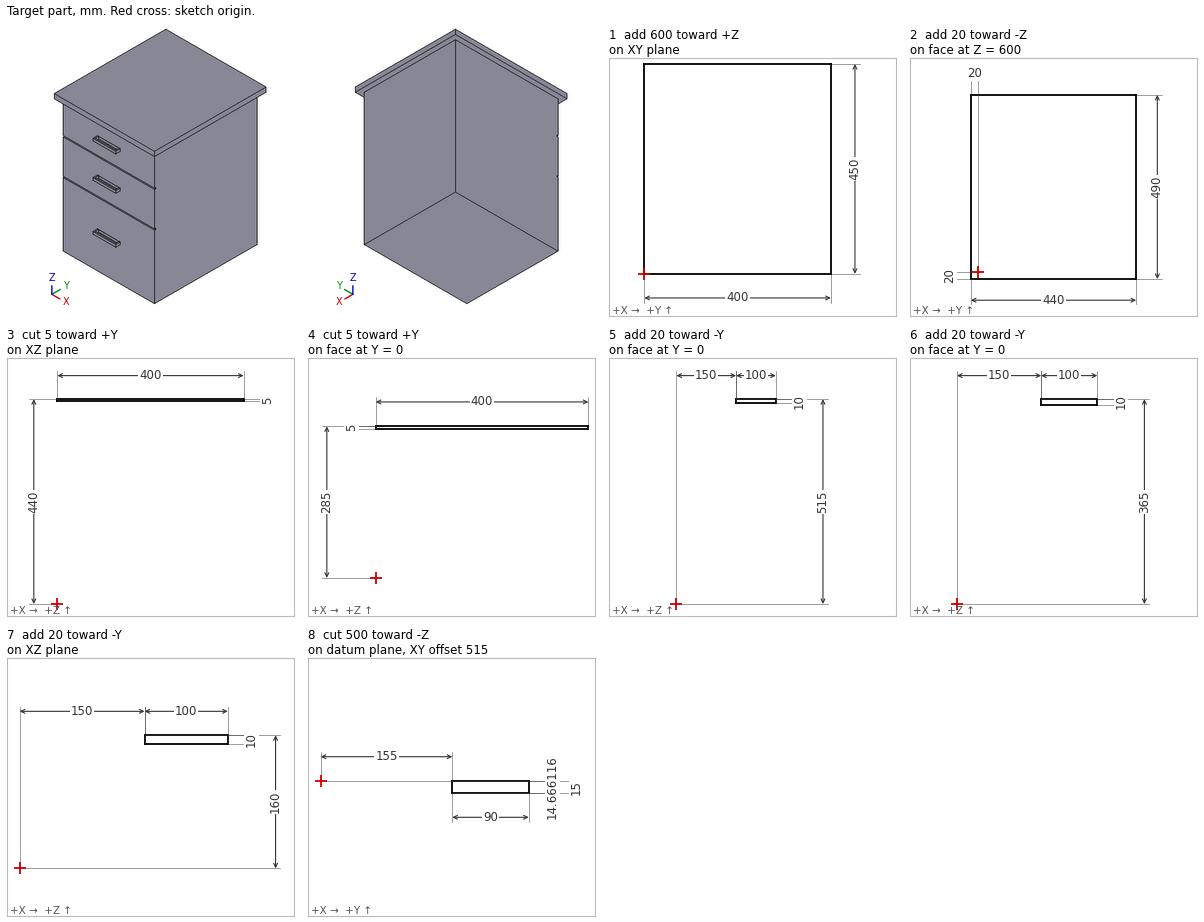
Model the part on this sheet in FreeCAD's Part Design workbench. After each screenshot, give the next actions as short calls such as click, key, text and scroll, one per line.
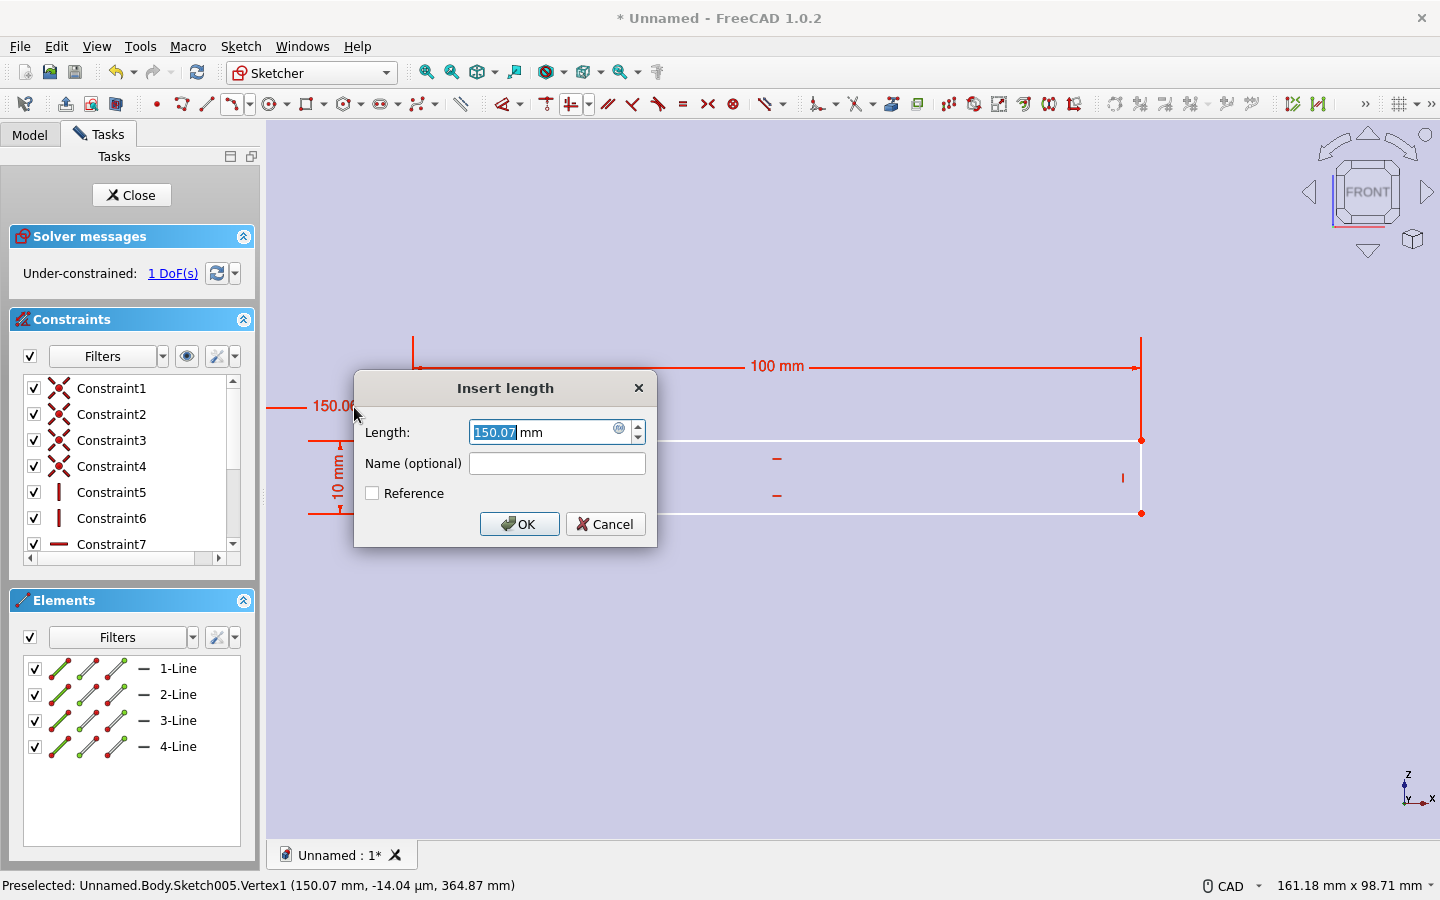
text(150)
key(Return)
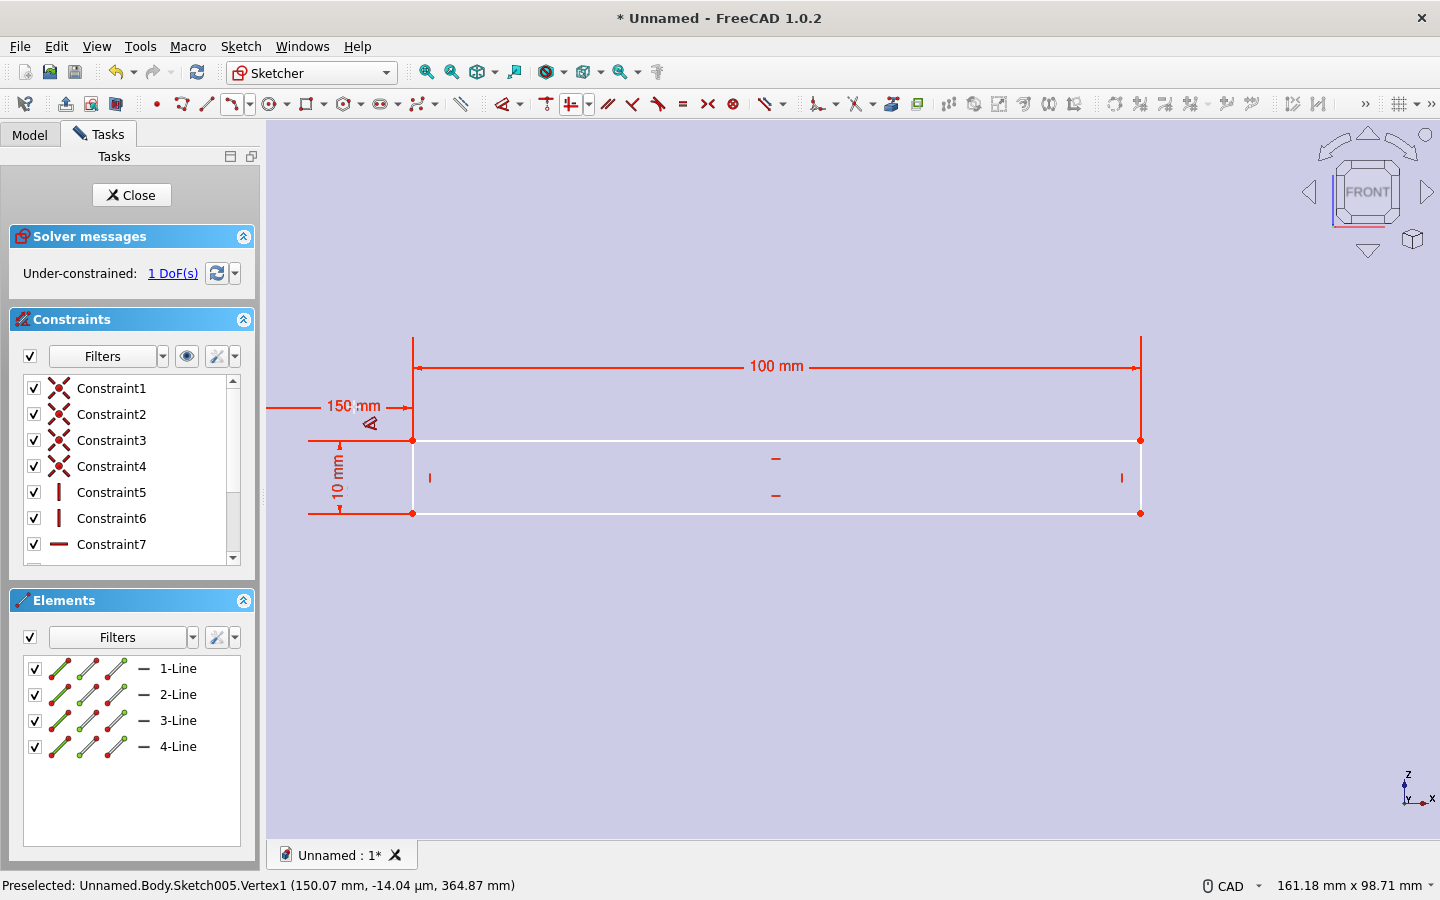
click(413, 441)
click(447, 626)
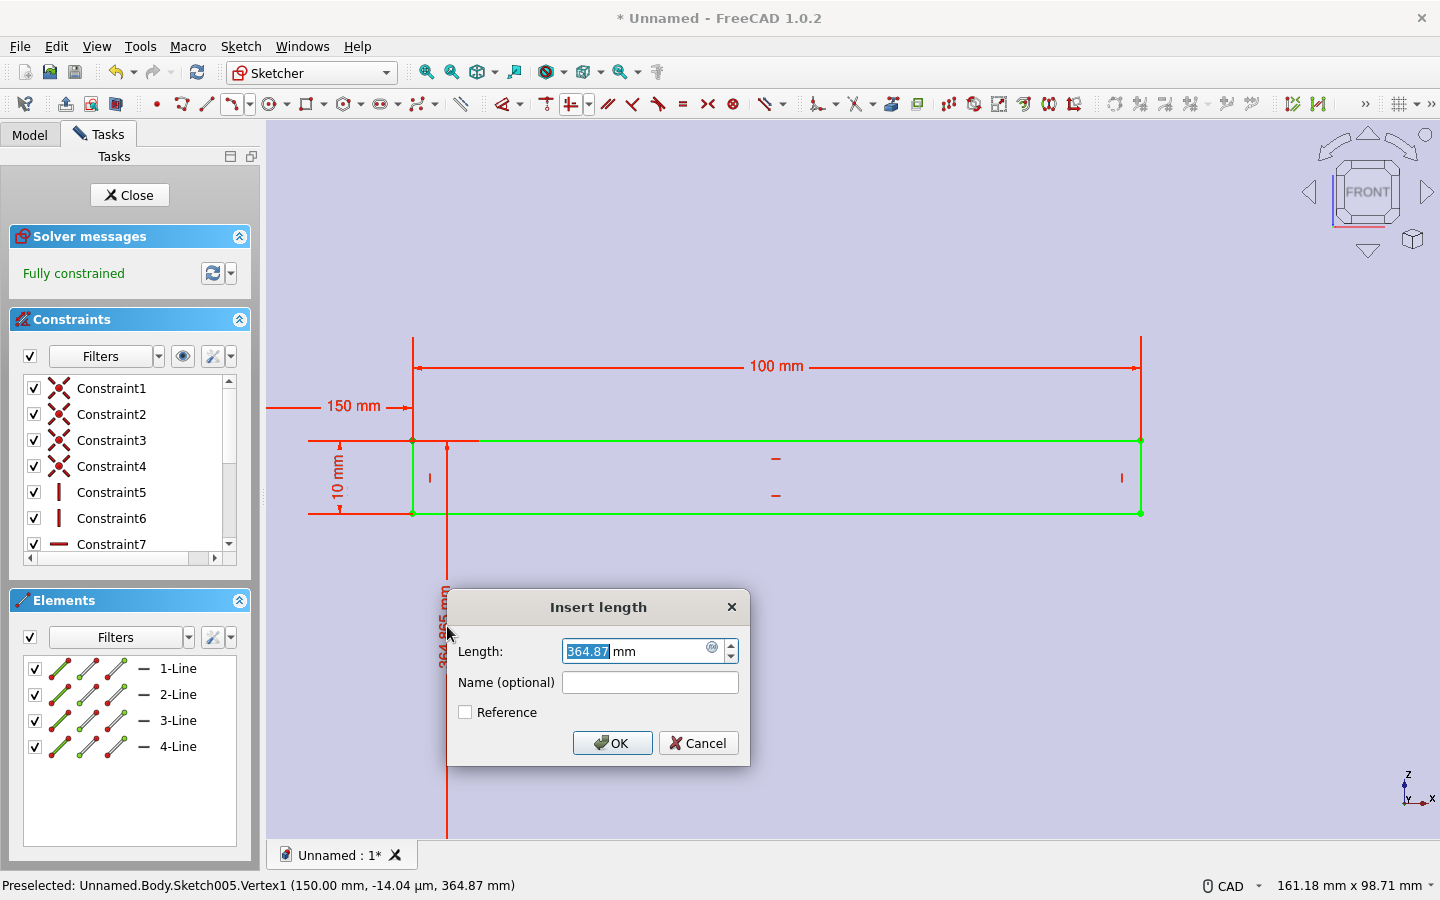
text(365)
key(Return)
key(Escape)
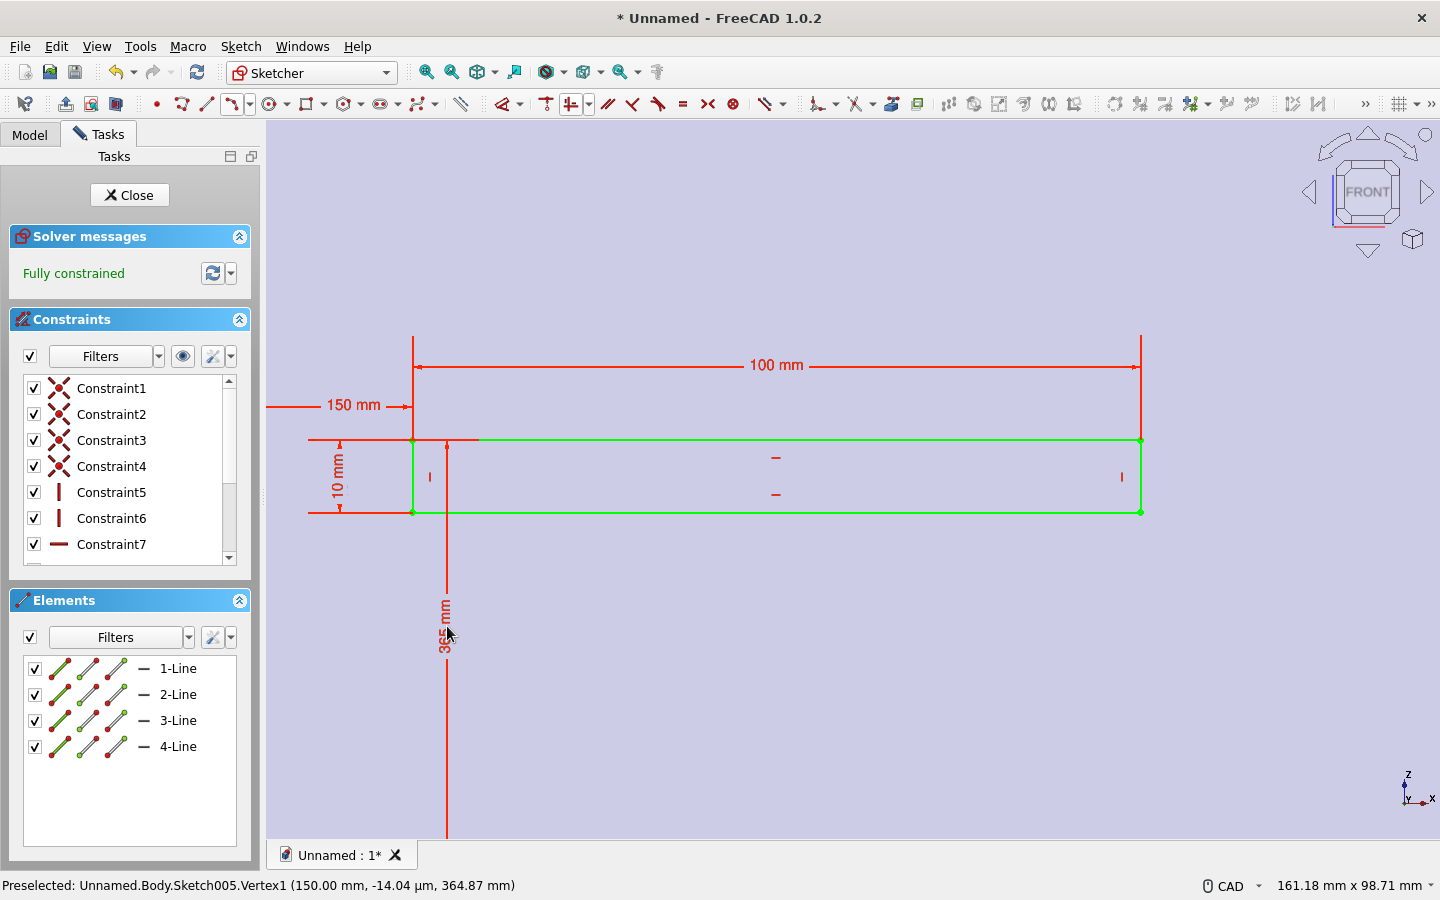
click(130, 195)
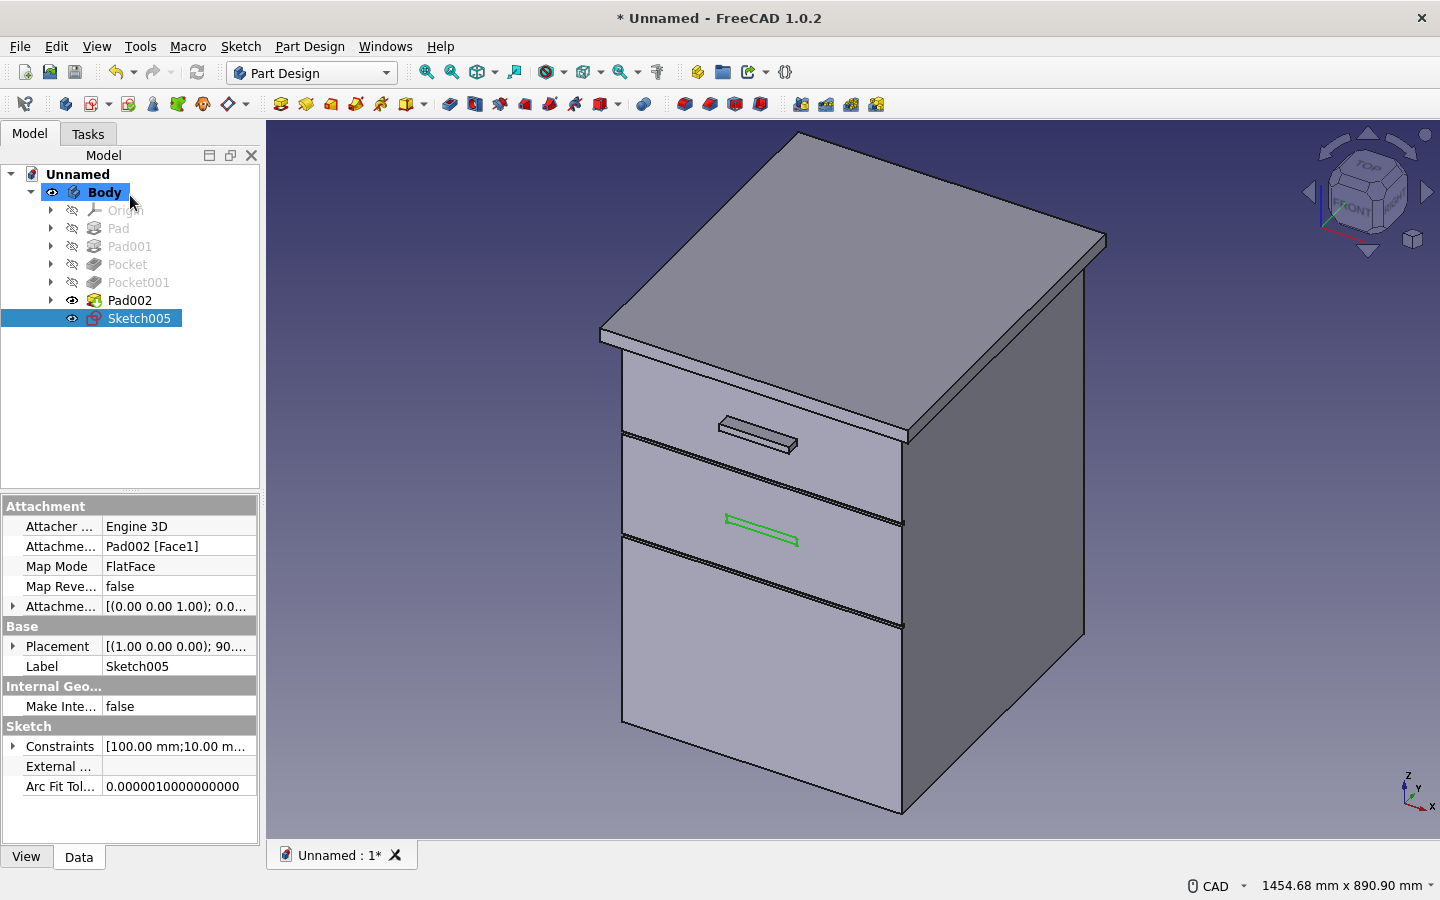
click(281, 104)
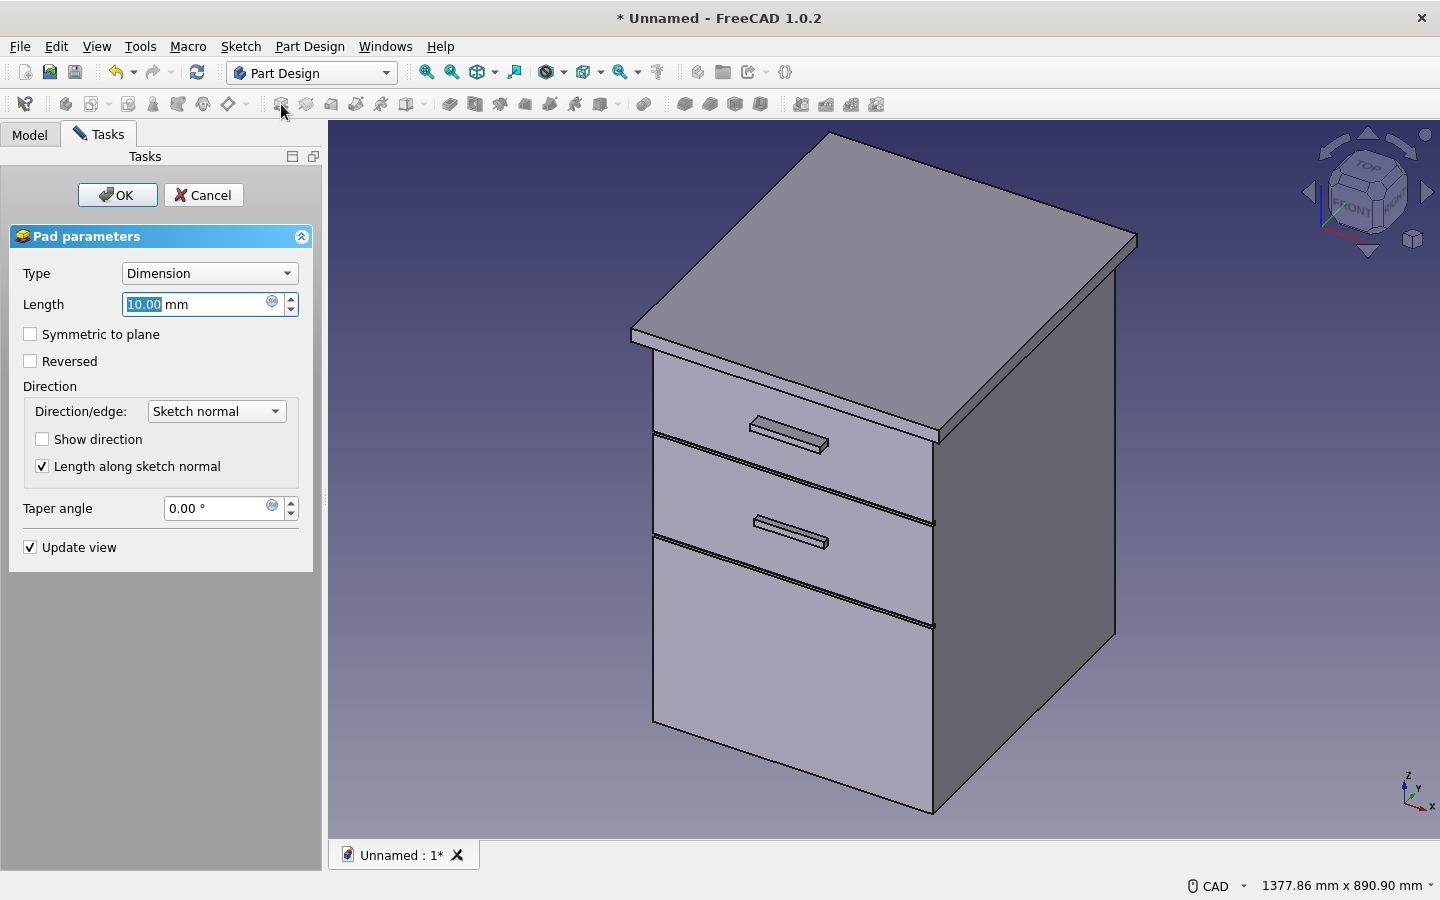
text(20)
key(Tab)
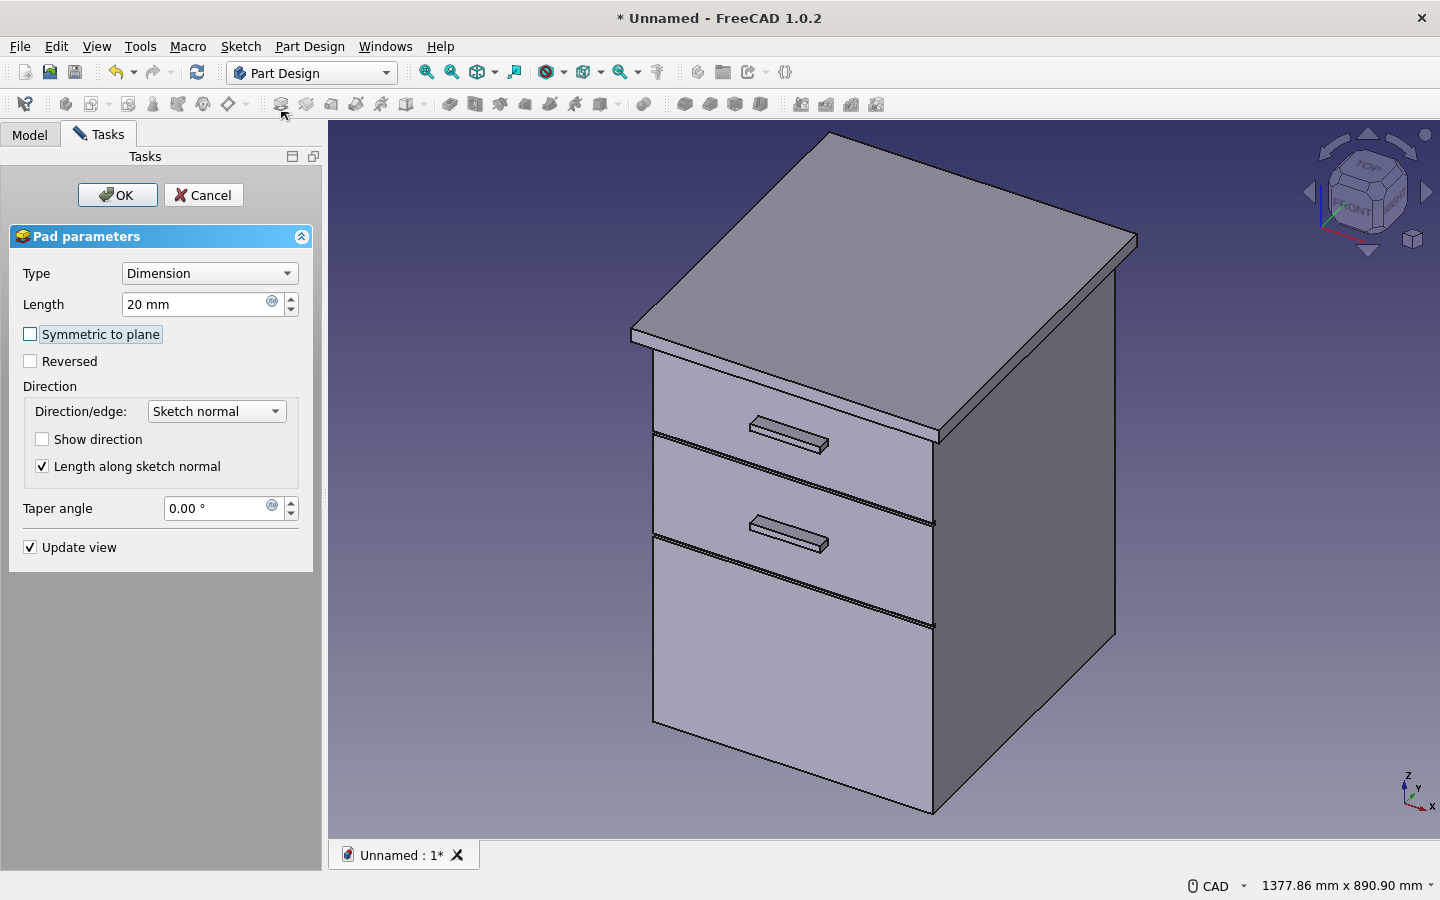
click(118, 195)